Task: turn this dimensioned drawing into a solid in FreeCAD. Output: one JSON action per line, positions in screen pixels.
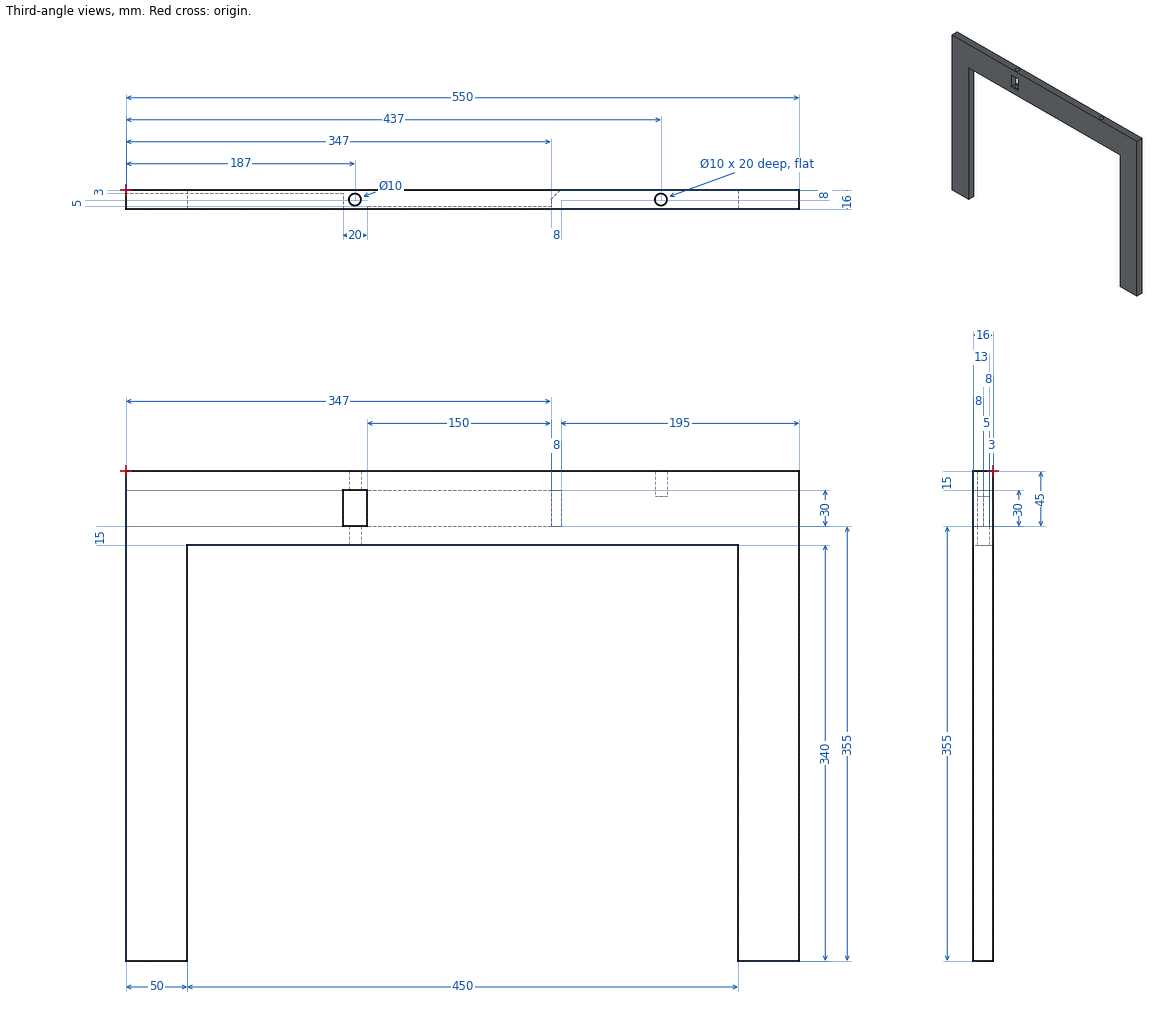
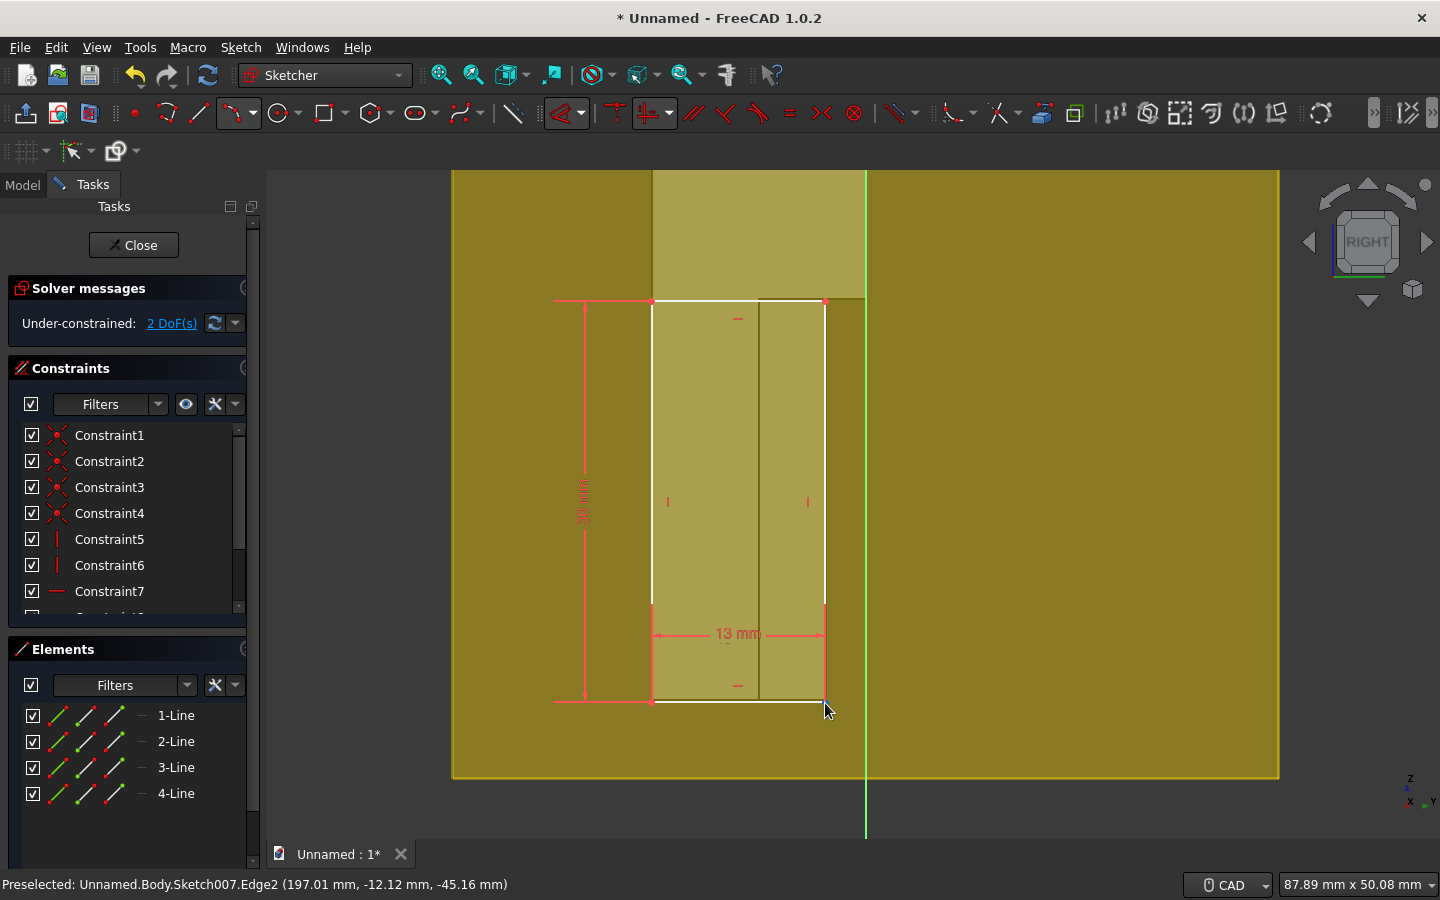
{"action": "left_click", "coordinate": [825, 702]}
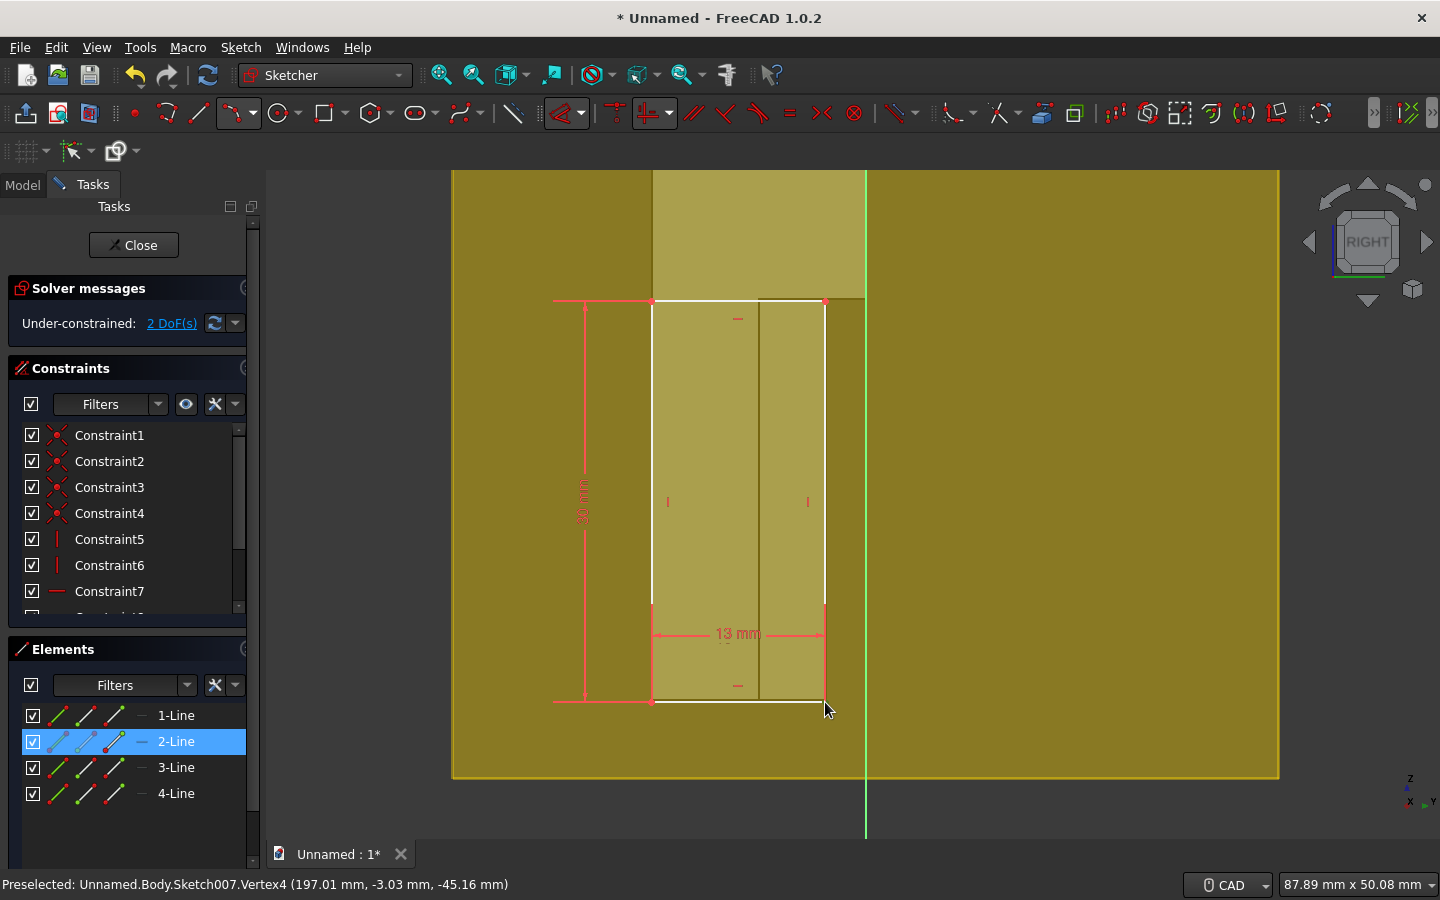
{"action": "left_click", "coordinate": [584, 114]}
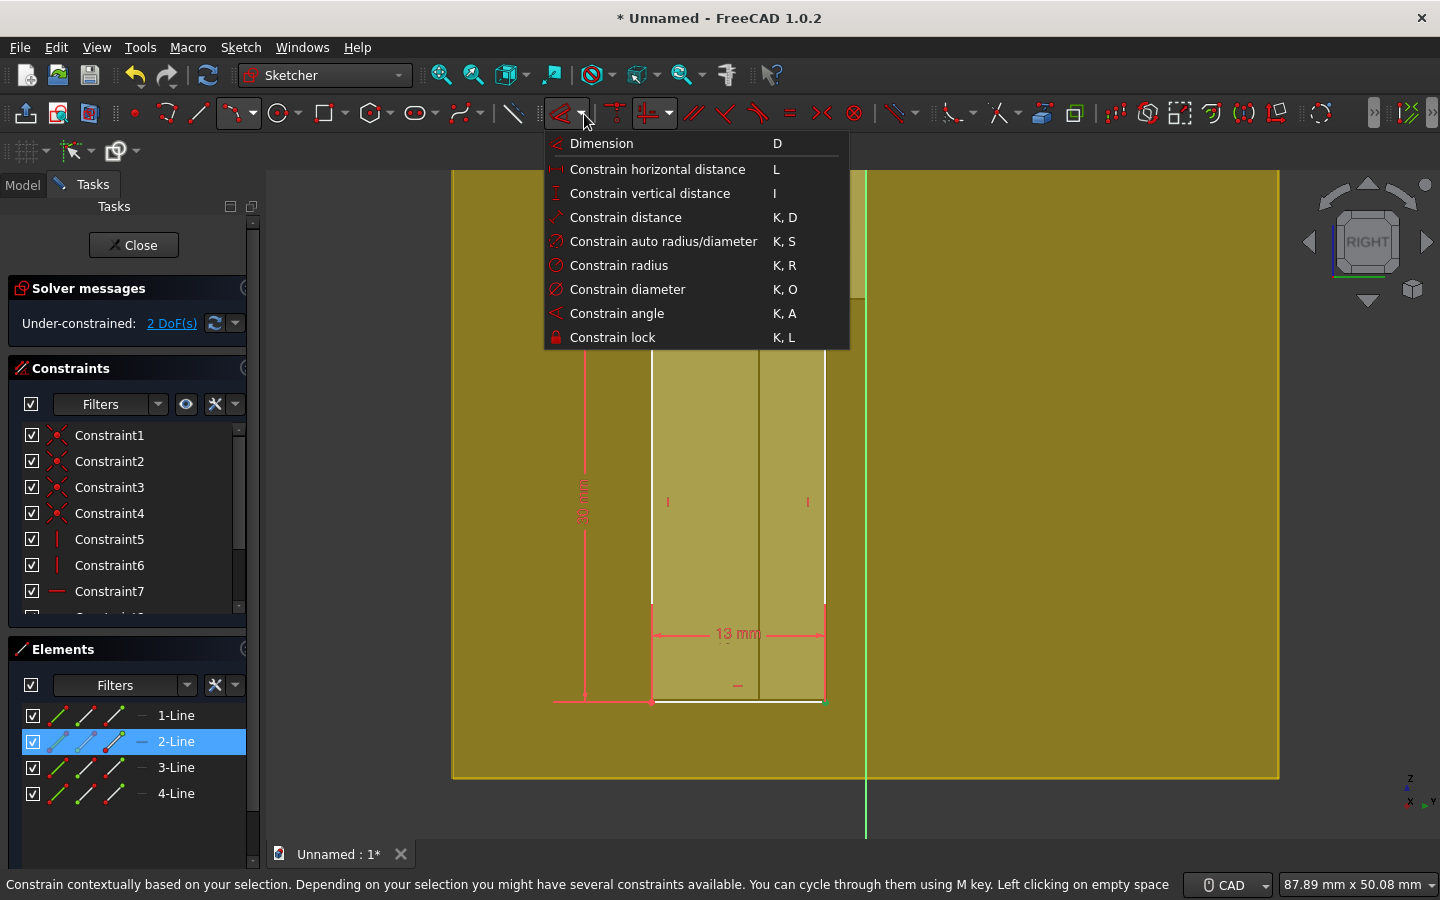
{"action": "left_click", "coordinate": [697, 169]}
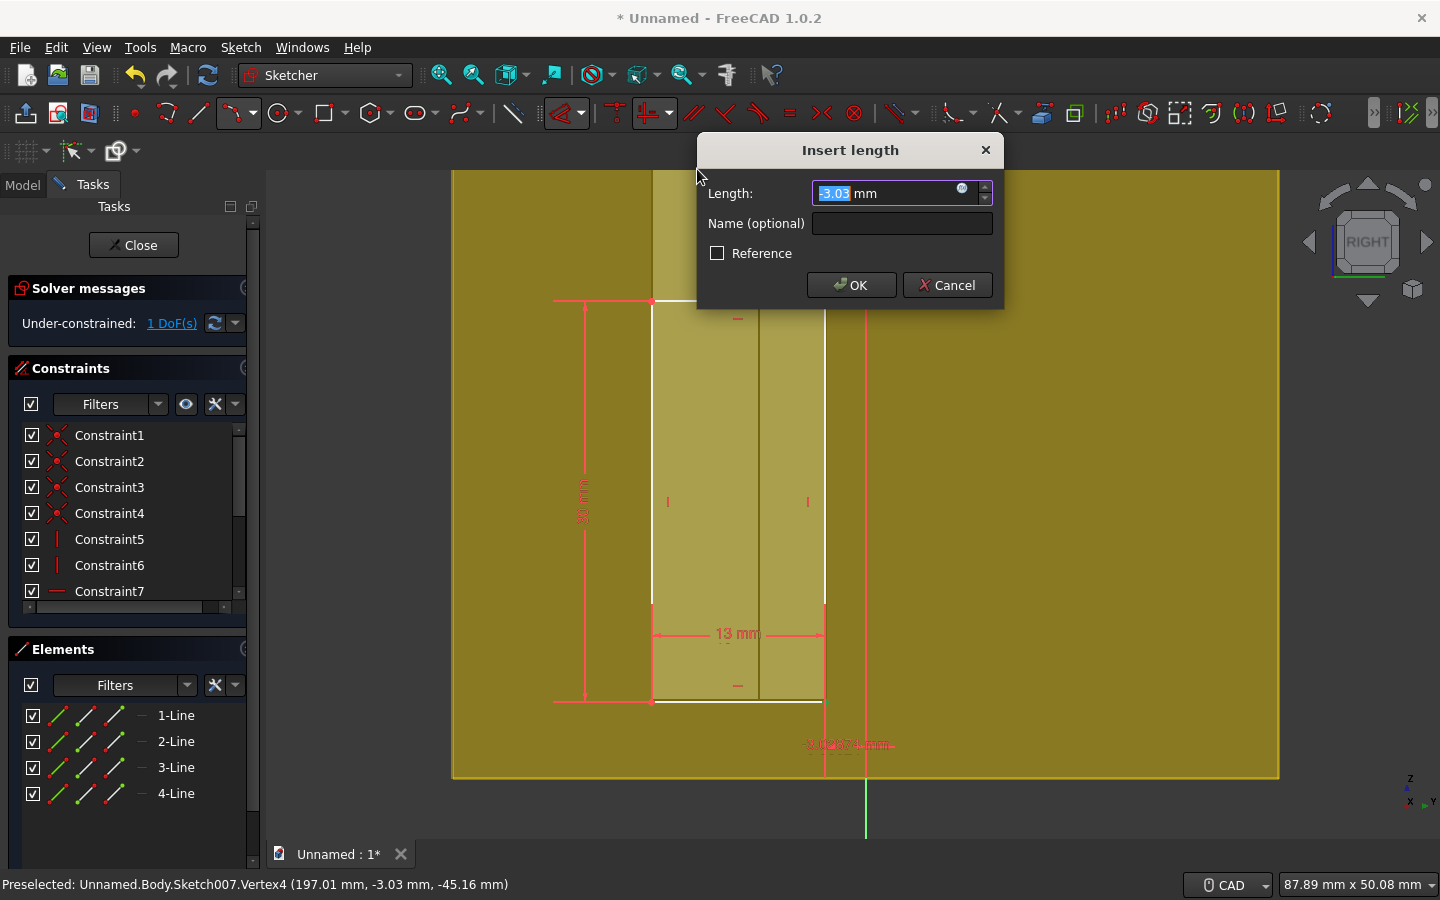
{"action": "type", "text": "-3"}
{"action": "key", "text": "Return"}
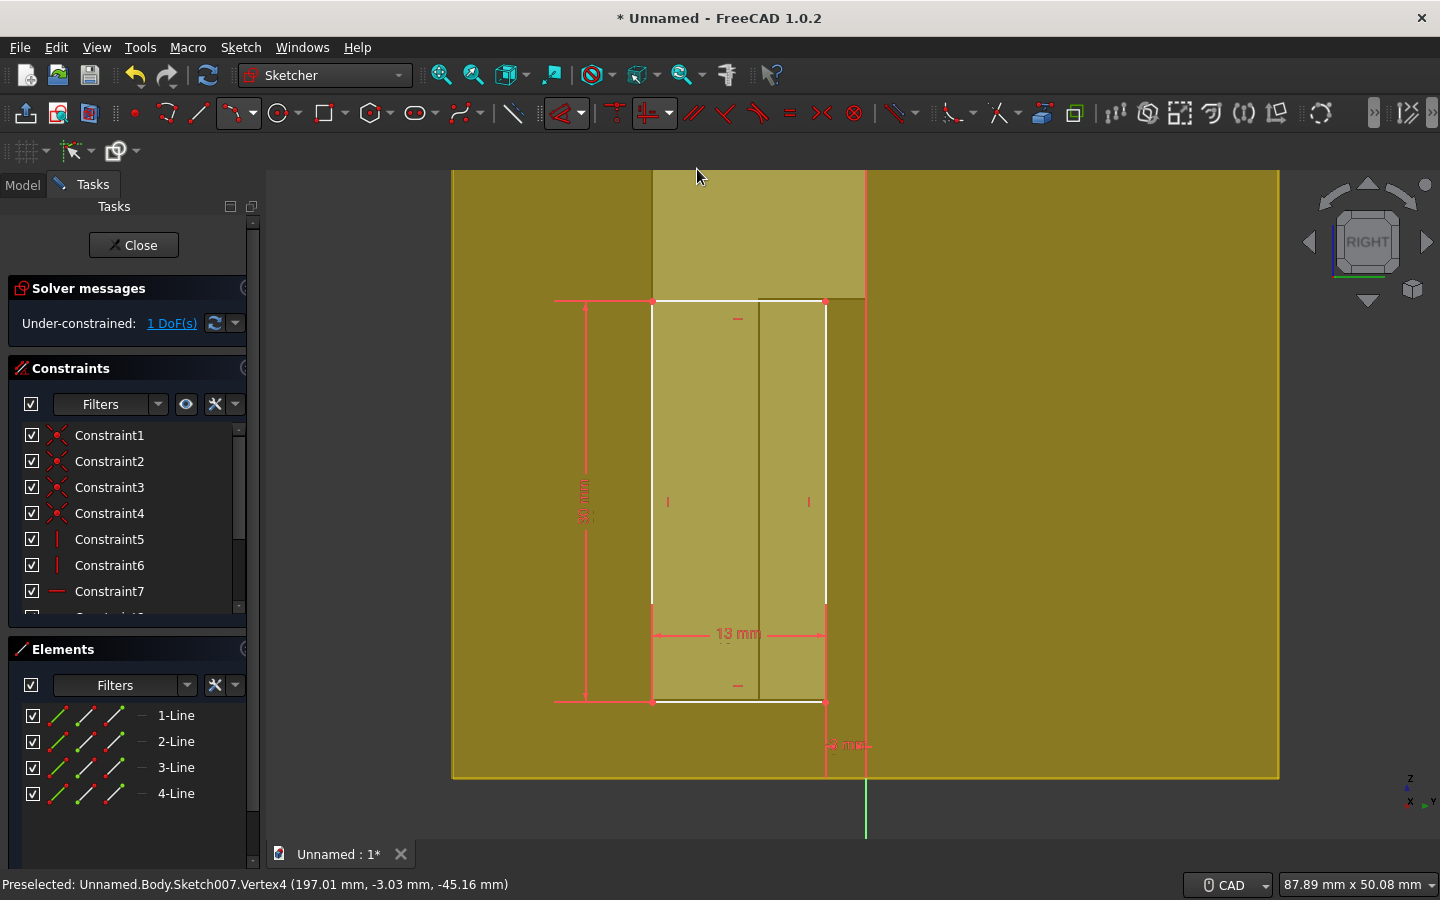
{"action": "left_click", "coordinate": [652, 301]}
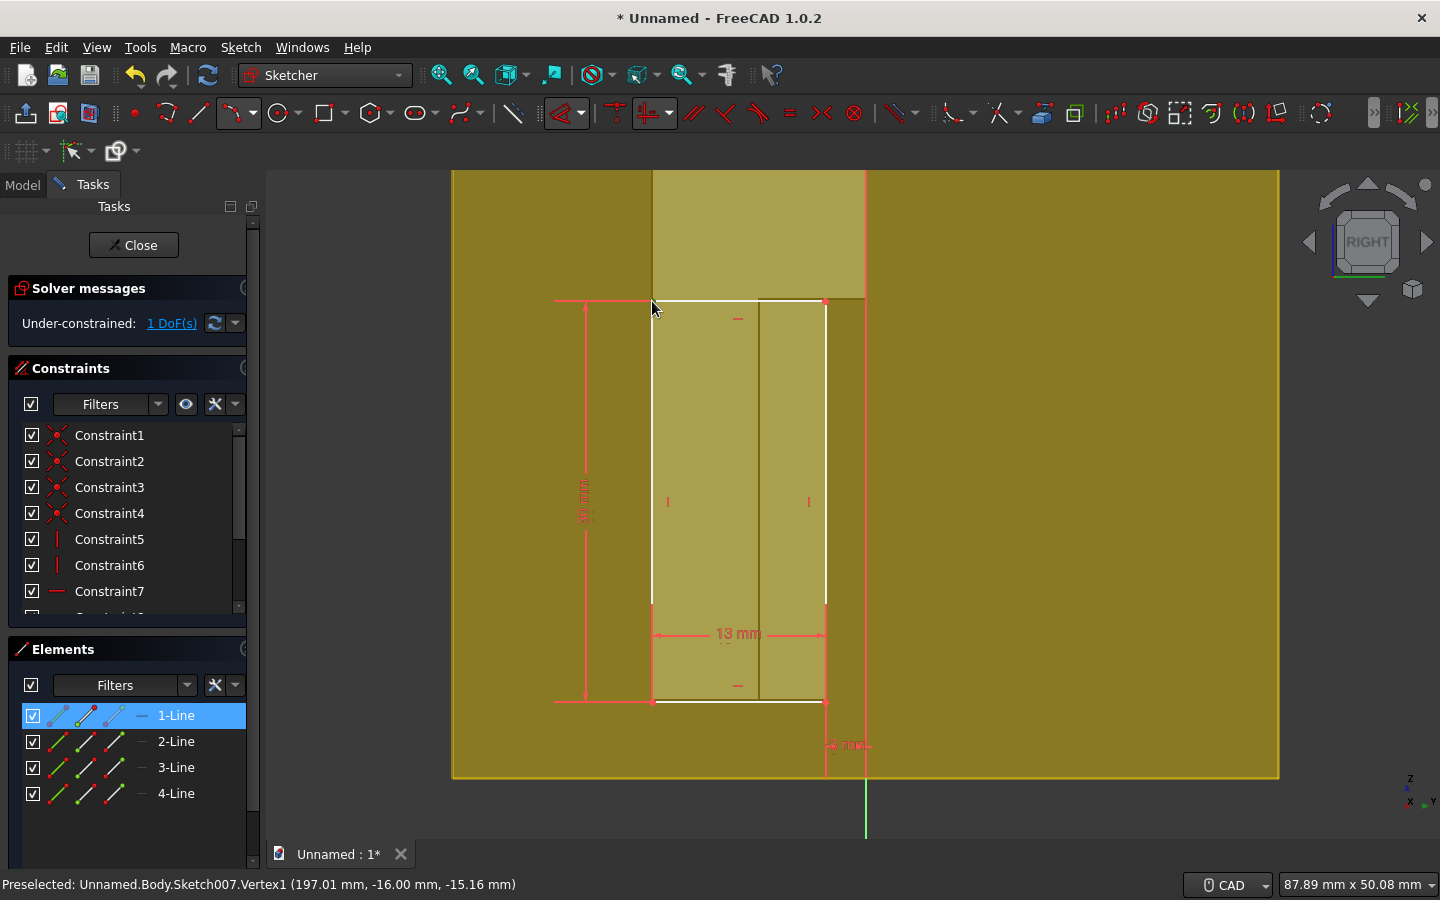
{"action": "left_click", "coordinate": [584, 114]}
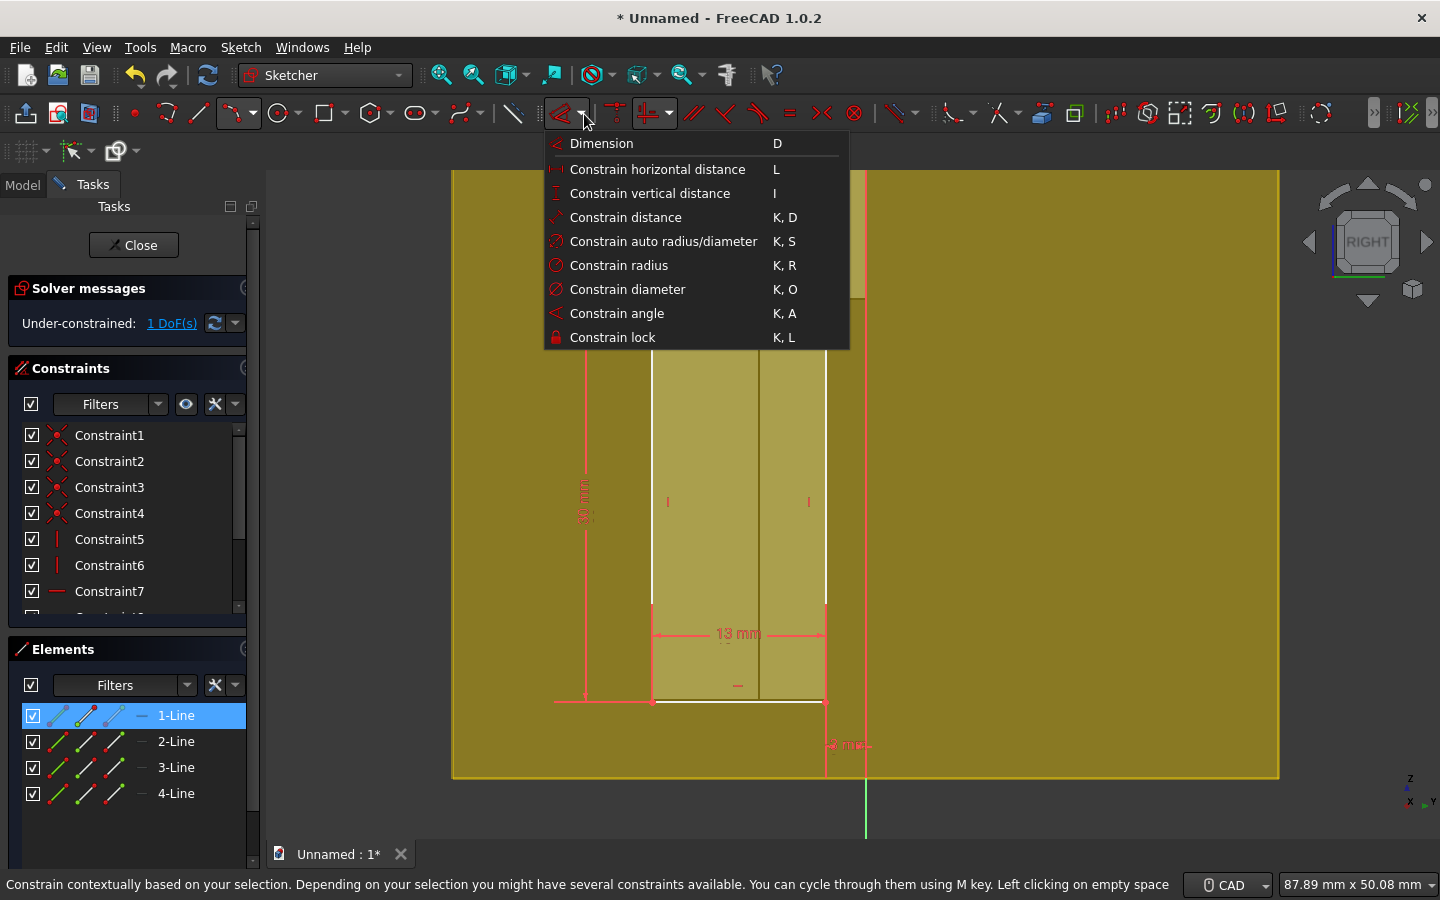
{"action": "left_click", "coordinate": [697, 193]}